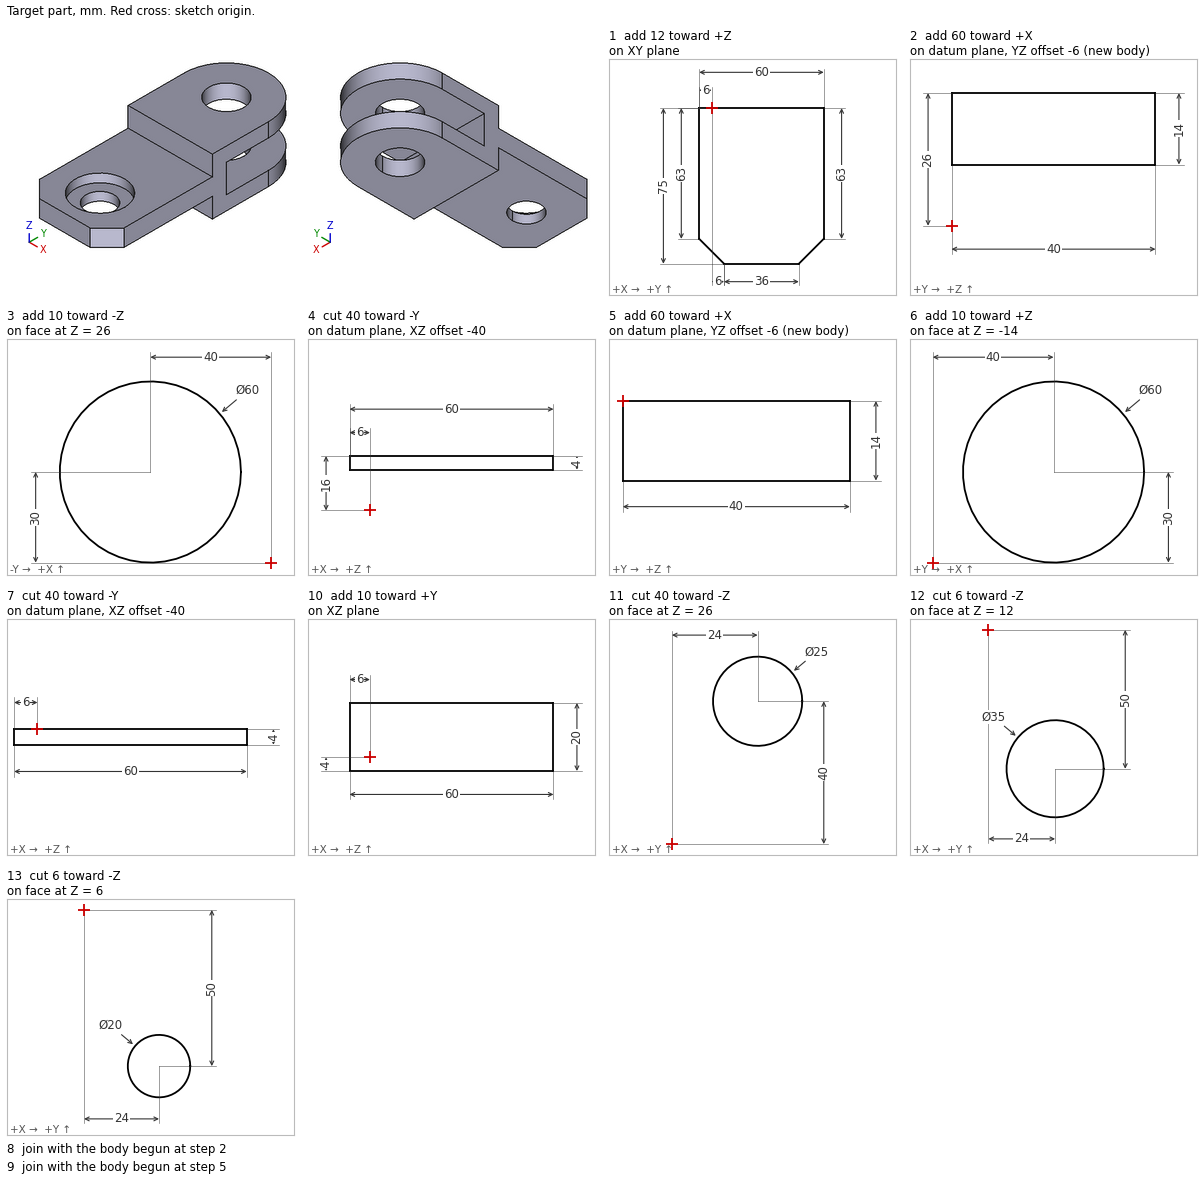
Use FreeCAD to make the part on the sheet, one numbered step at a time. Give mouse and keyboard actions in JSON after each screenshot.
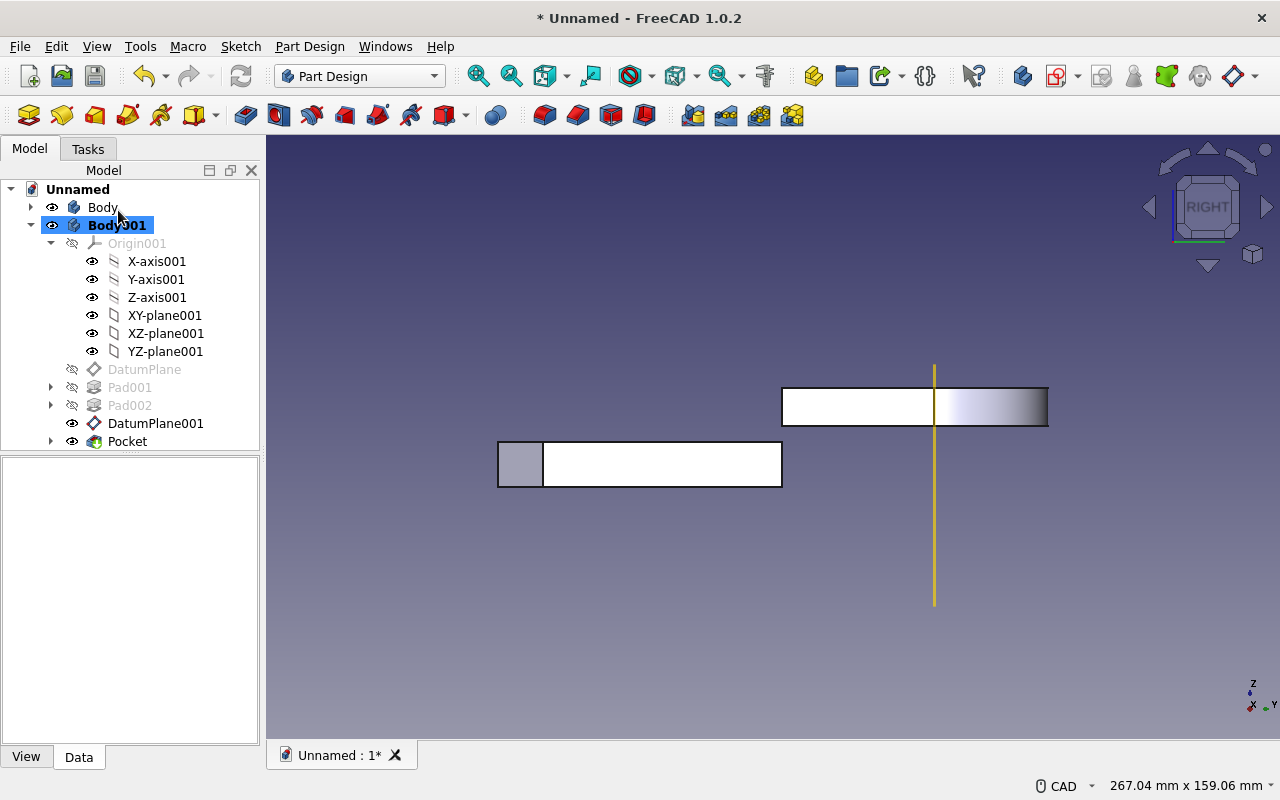
{"action": "left_click", "coordinate": [117, 423]}
{"action": "key", "text": "space"}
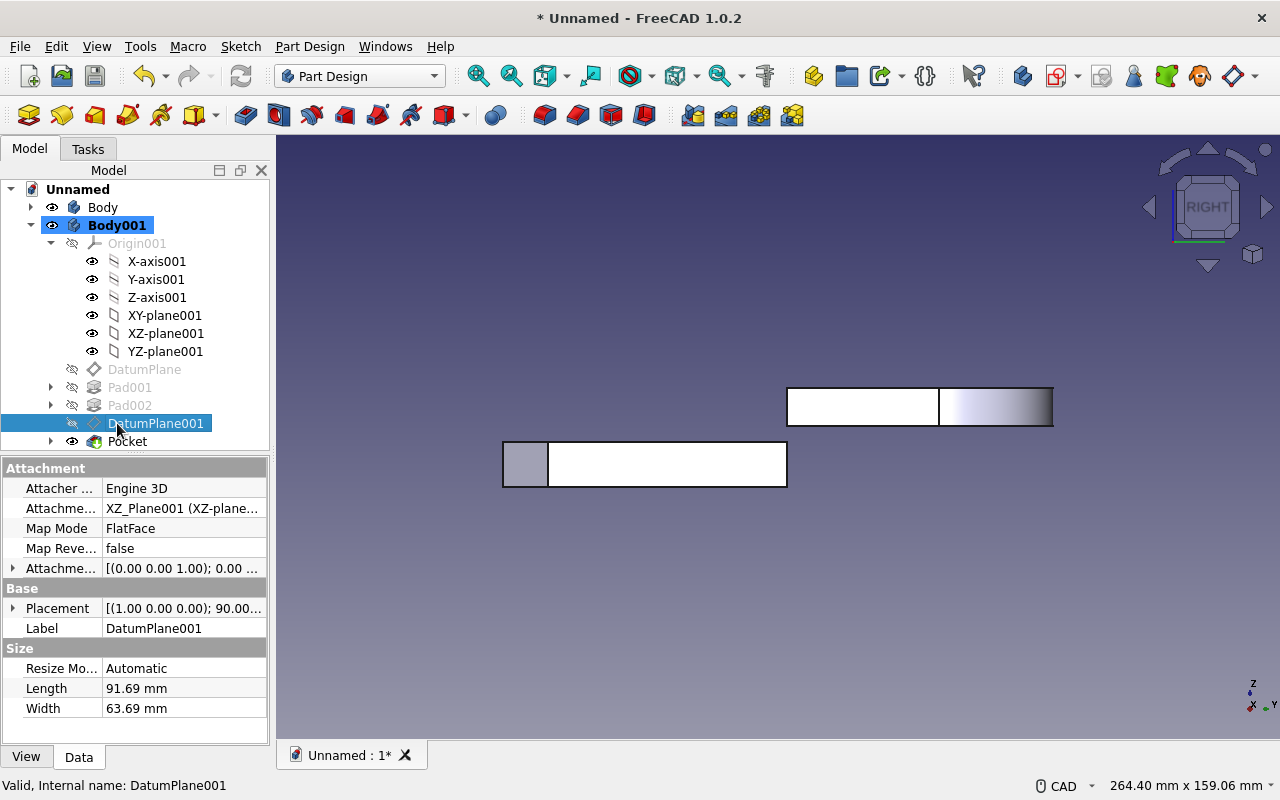
{"action": "left_click", "coordinate": [479, 76]}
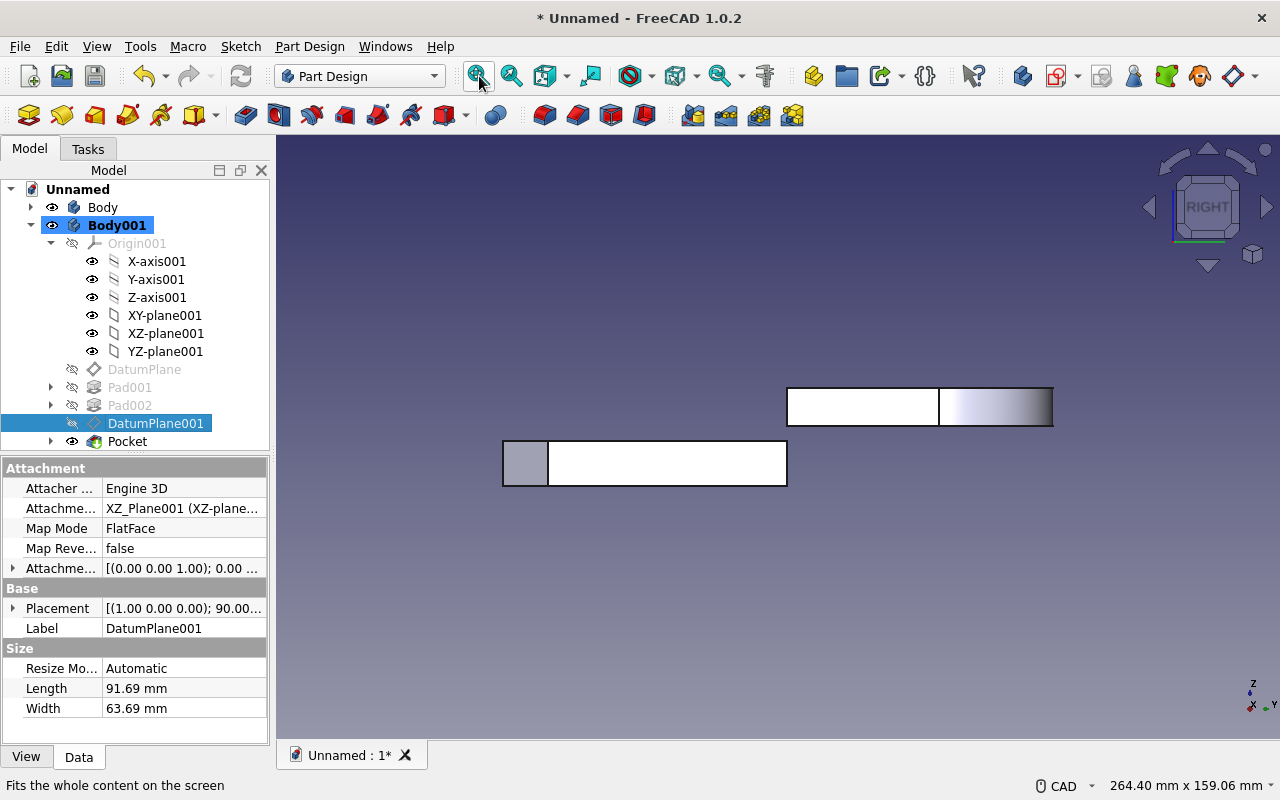
{"action": "left_click", "coordinate": [316, 699]}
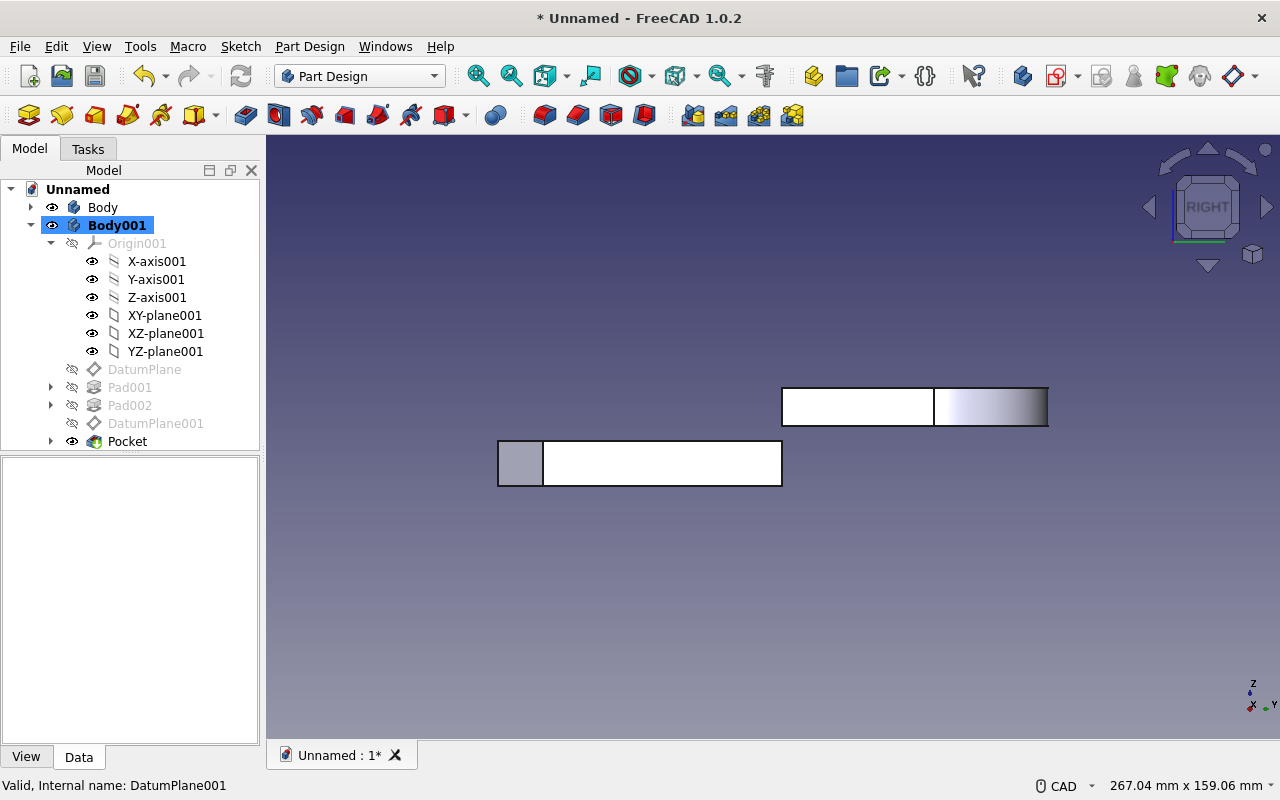
{"action": "left_click", "coordinate": [1023, 76]}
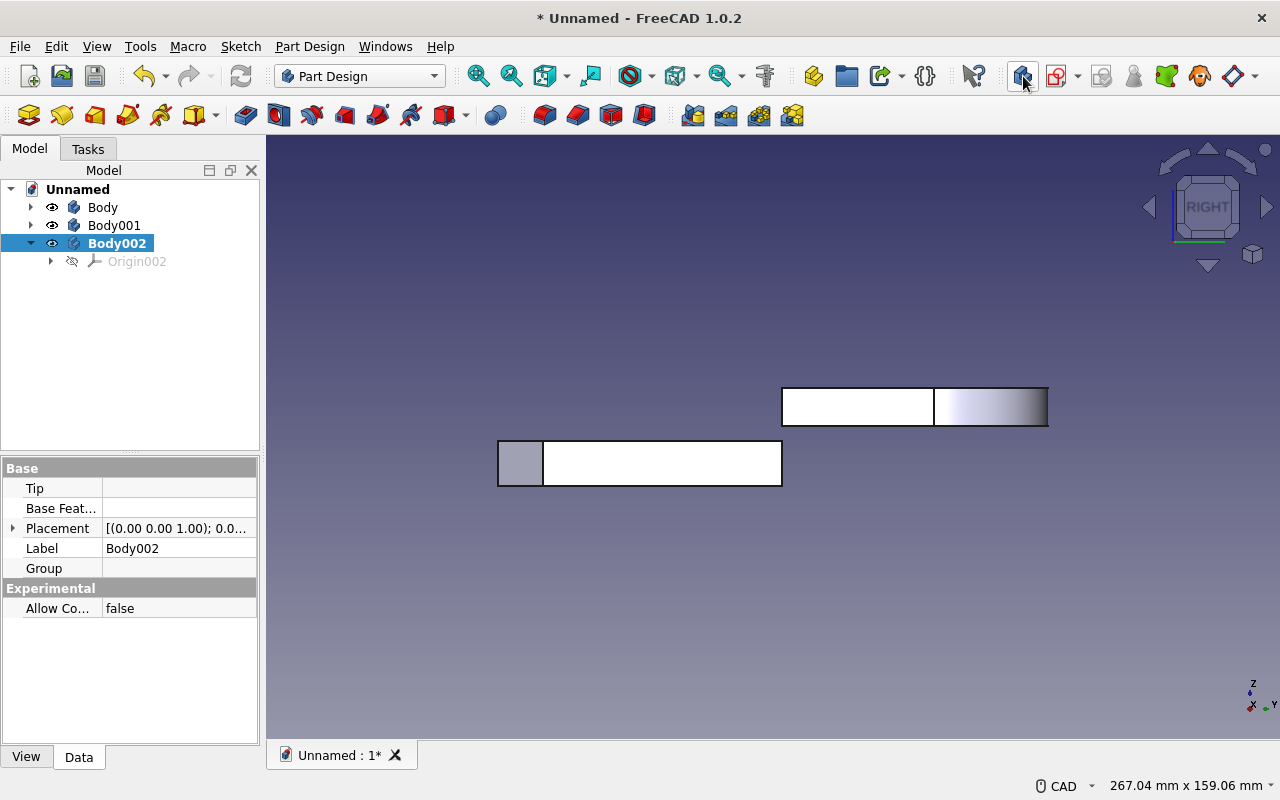
{"action": "left_click", "coordinate": [51, 261]}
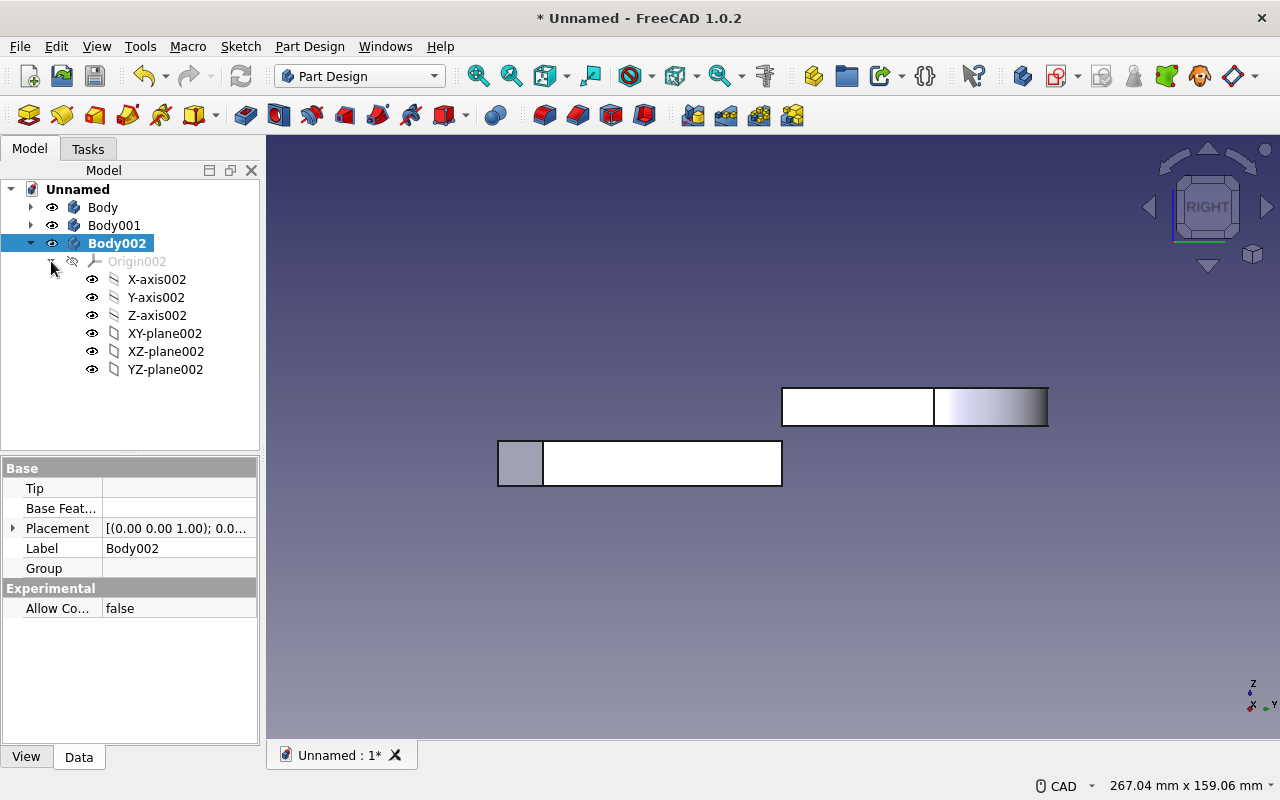
{"action": "left_click", "coordinate": [137, 369]}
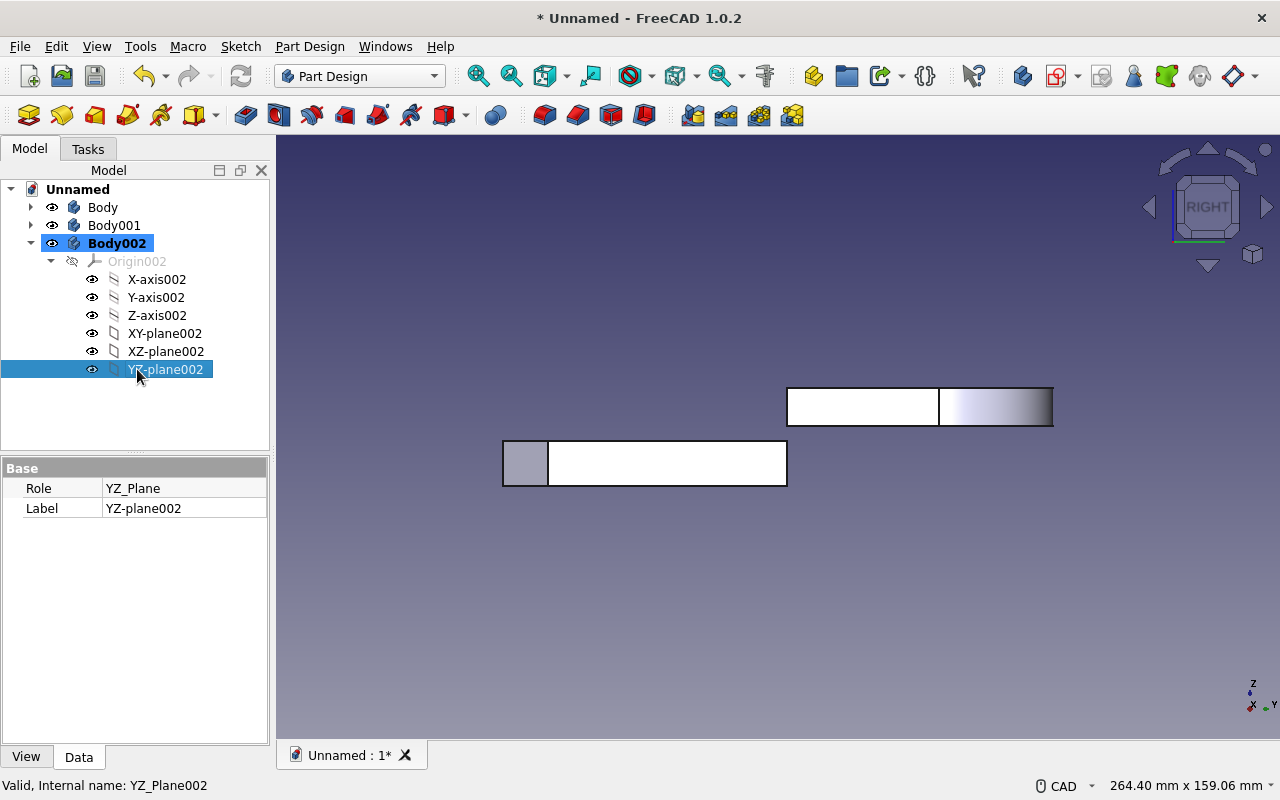
{"action": "left_click", "coordinate": [1232, 76]}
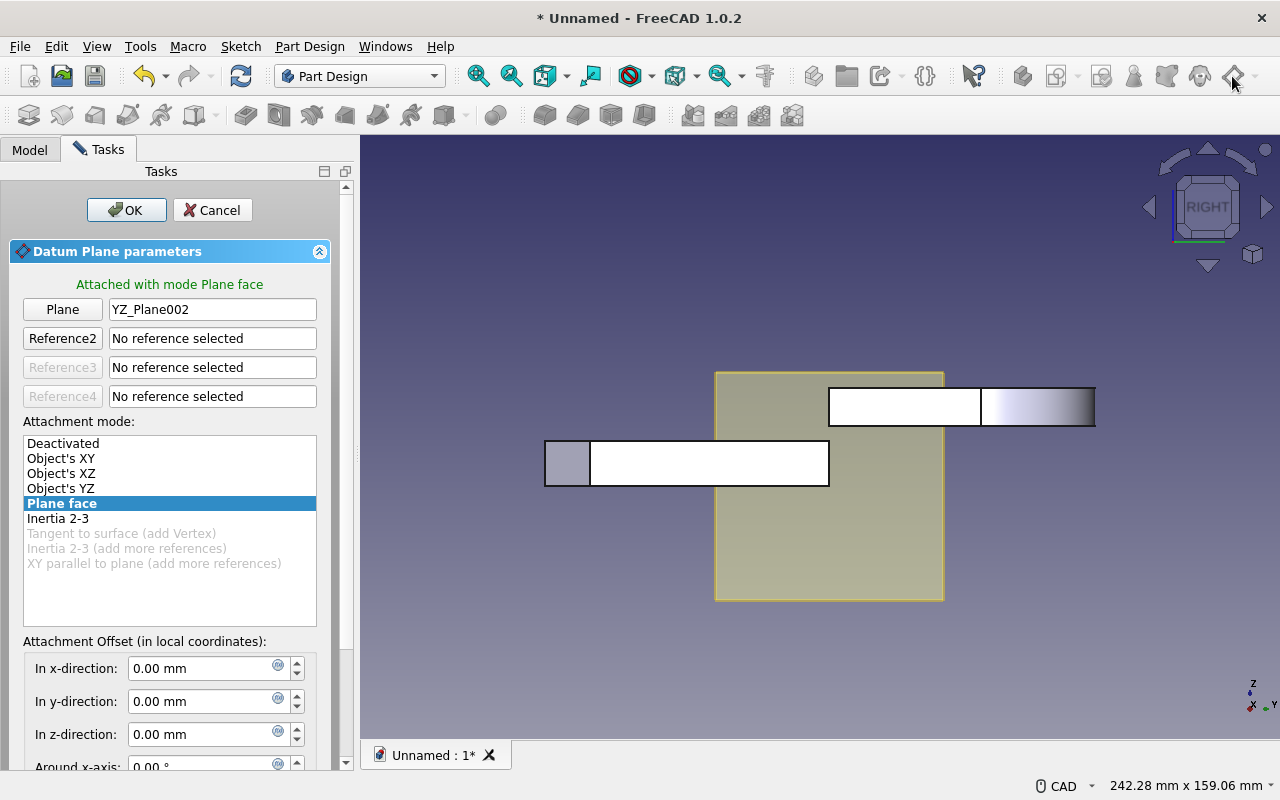
{"action": "triple_click", "coordinate": [210, 734]}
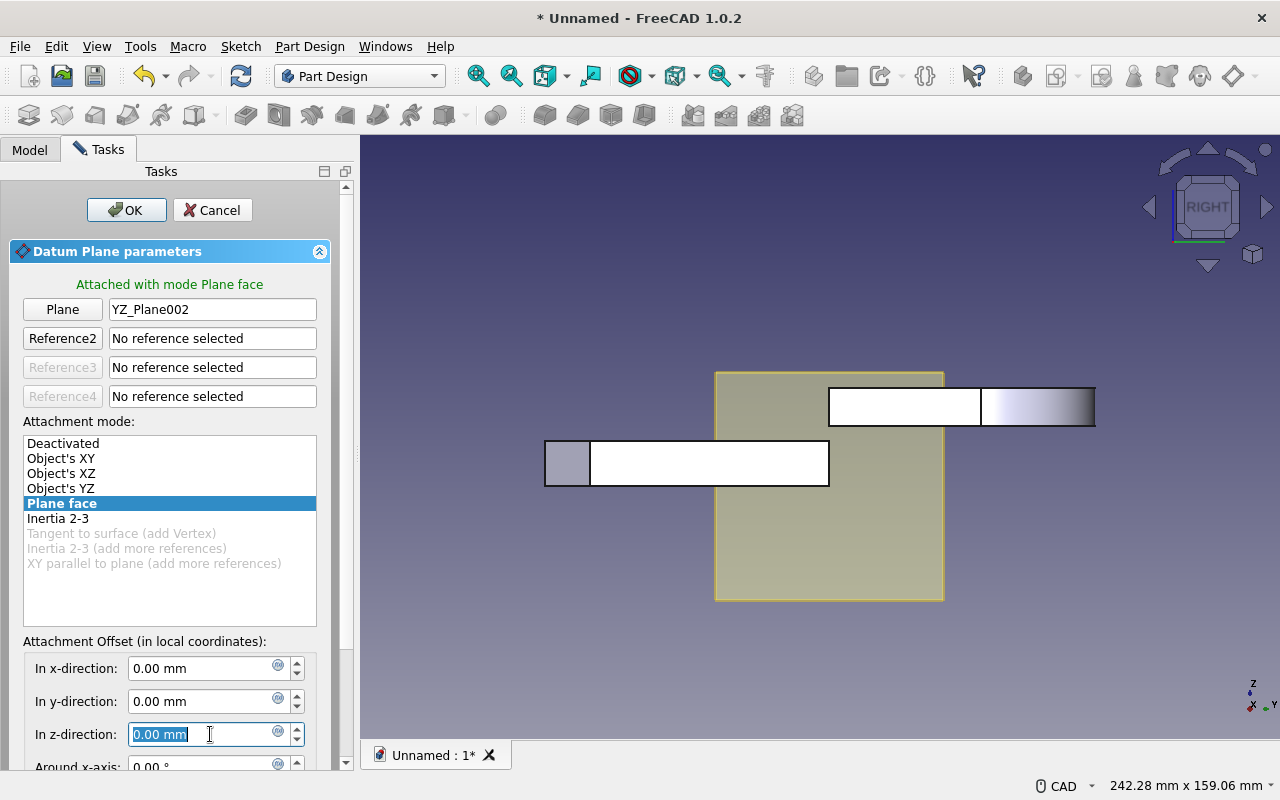
{"action": "type", "text": "-6"}
{"action": "key", "text": "Tab"}